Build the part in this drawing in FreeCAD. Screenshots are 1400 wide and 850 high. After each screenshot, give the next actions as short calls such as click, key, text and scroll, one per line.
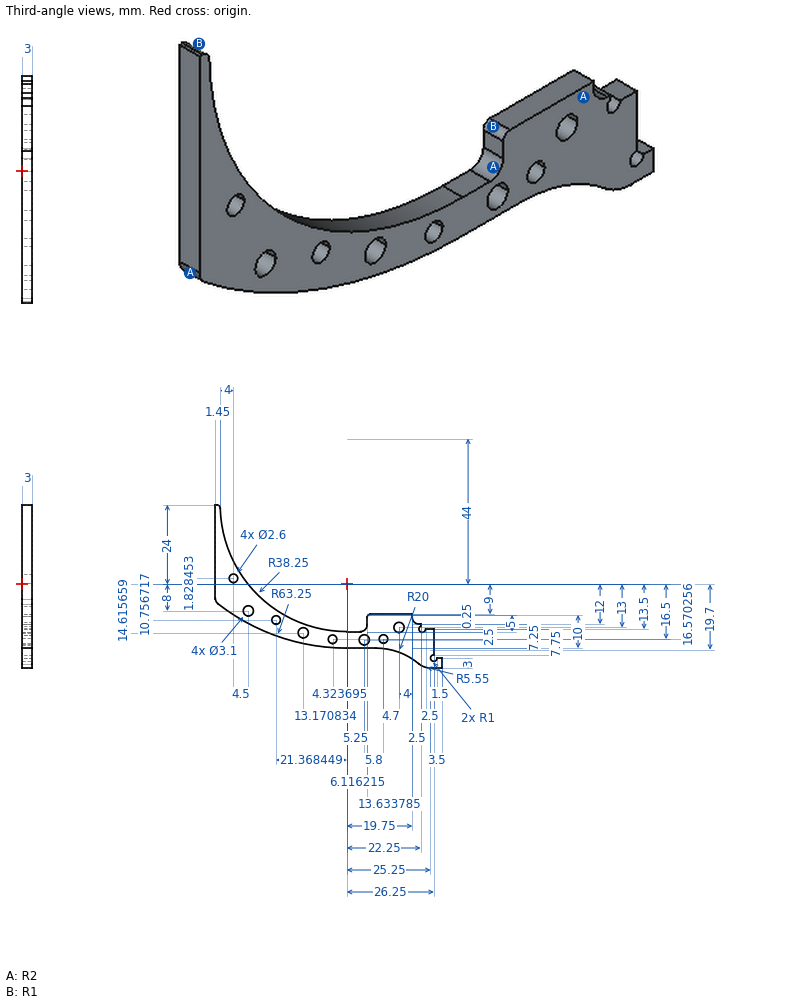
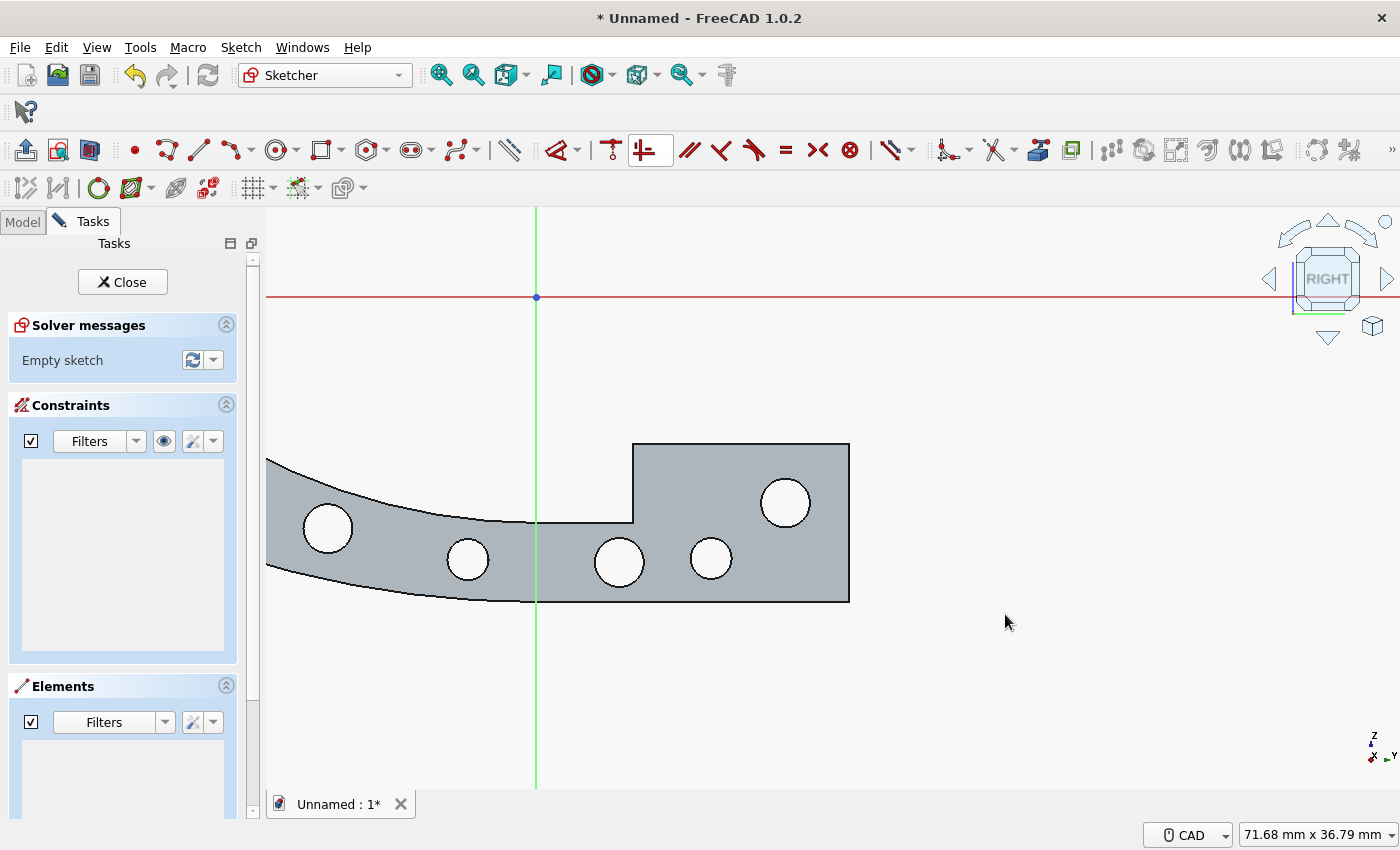
key(g)
key(r)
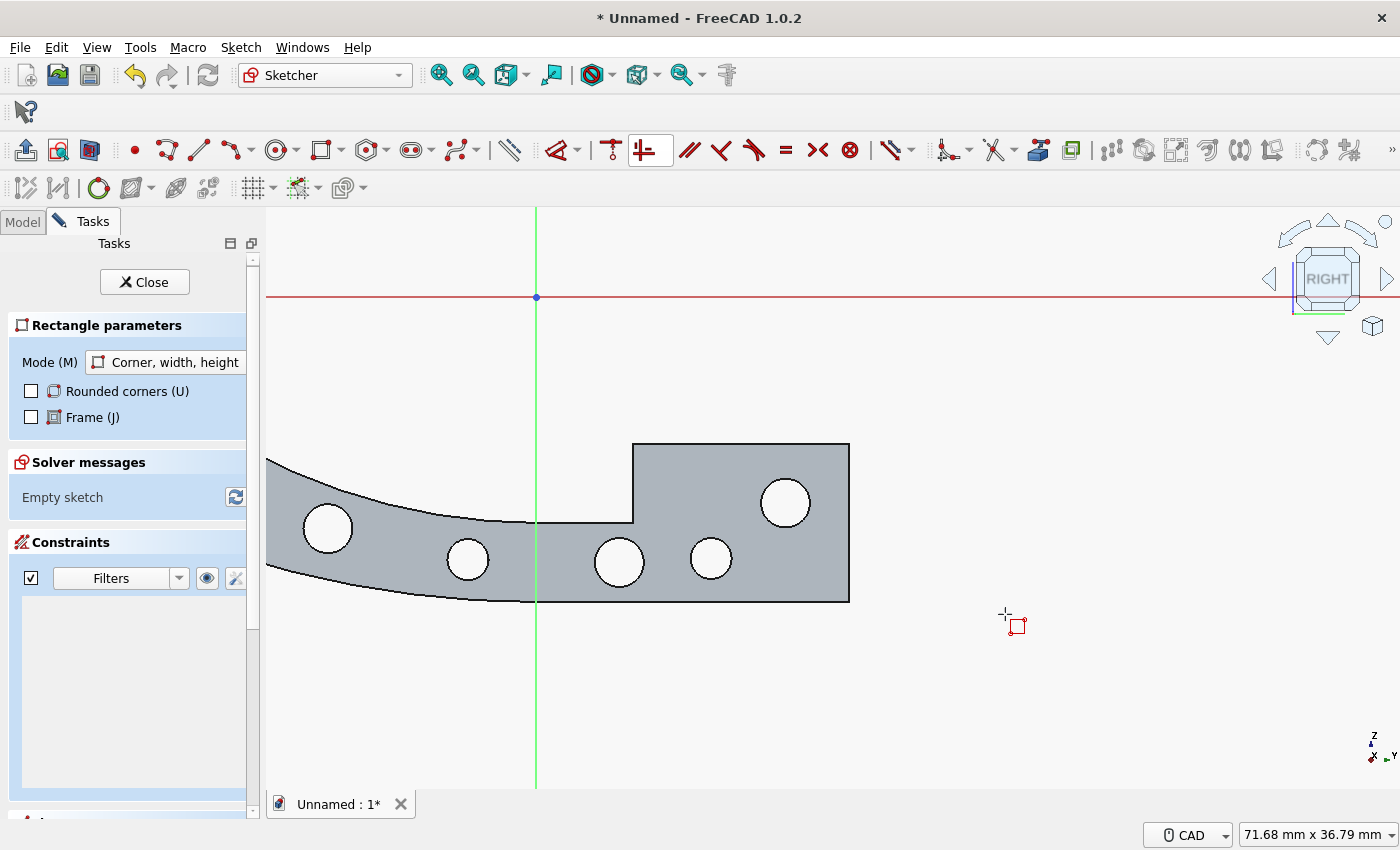
scroll(633, 440, up, 7)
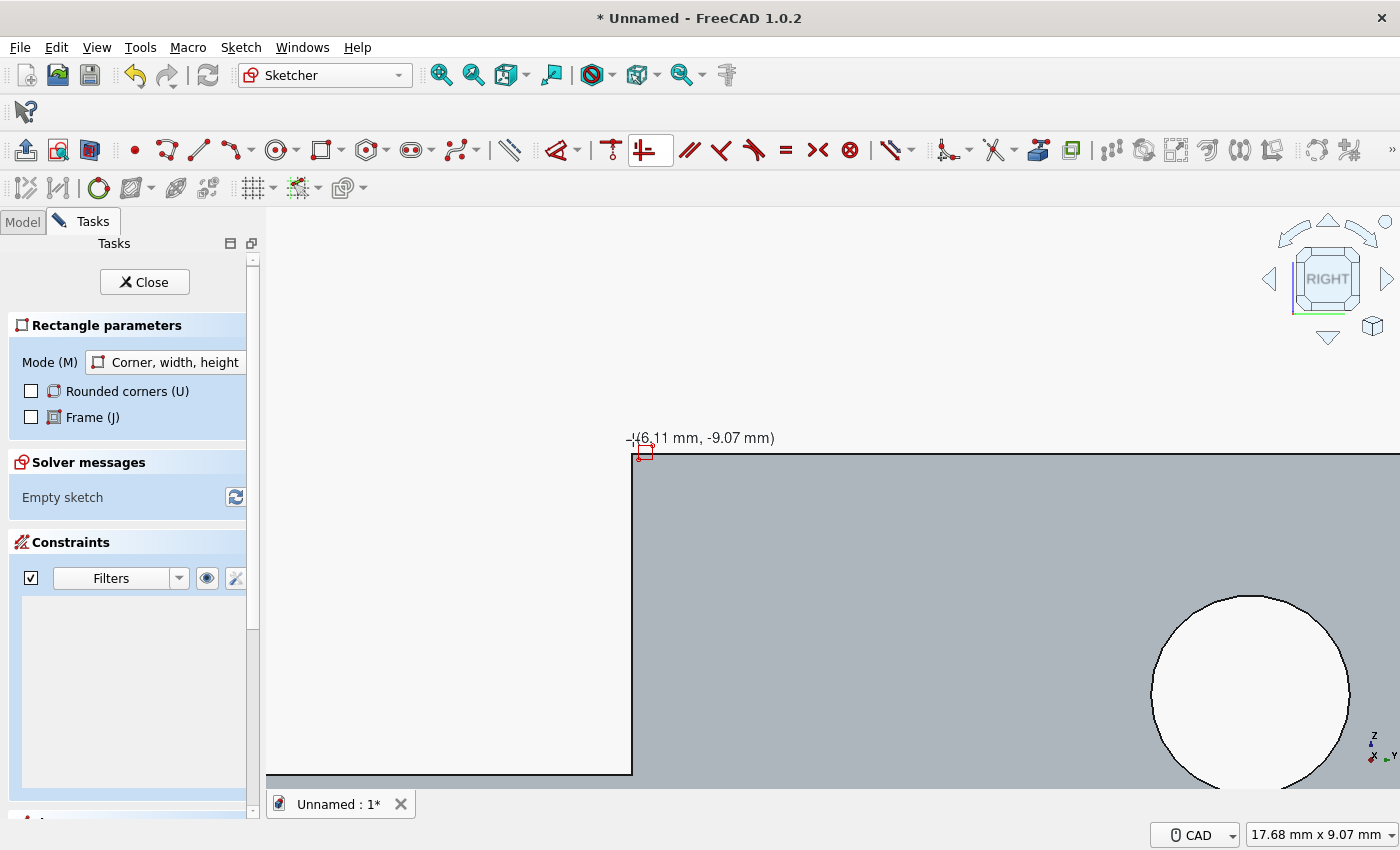
scroll(634, 441, down, 7)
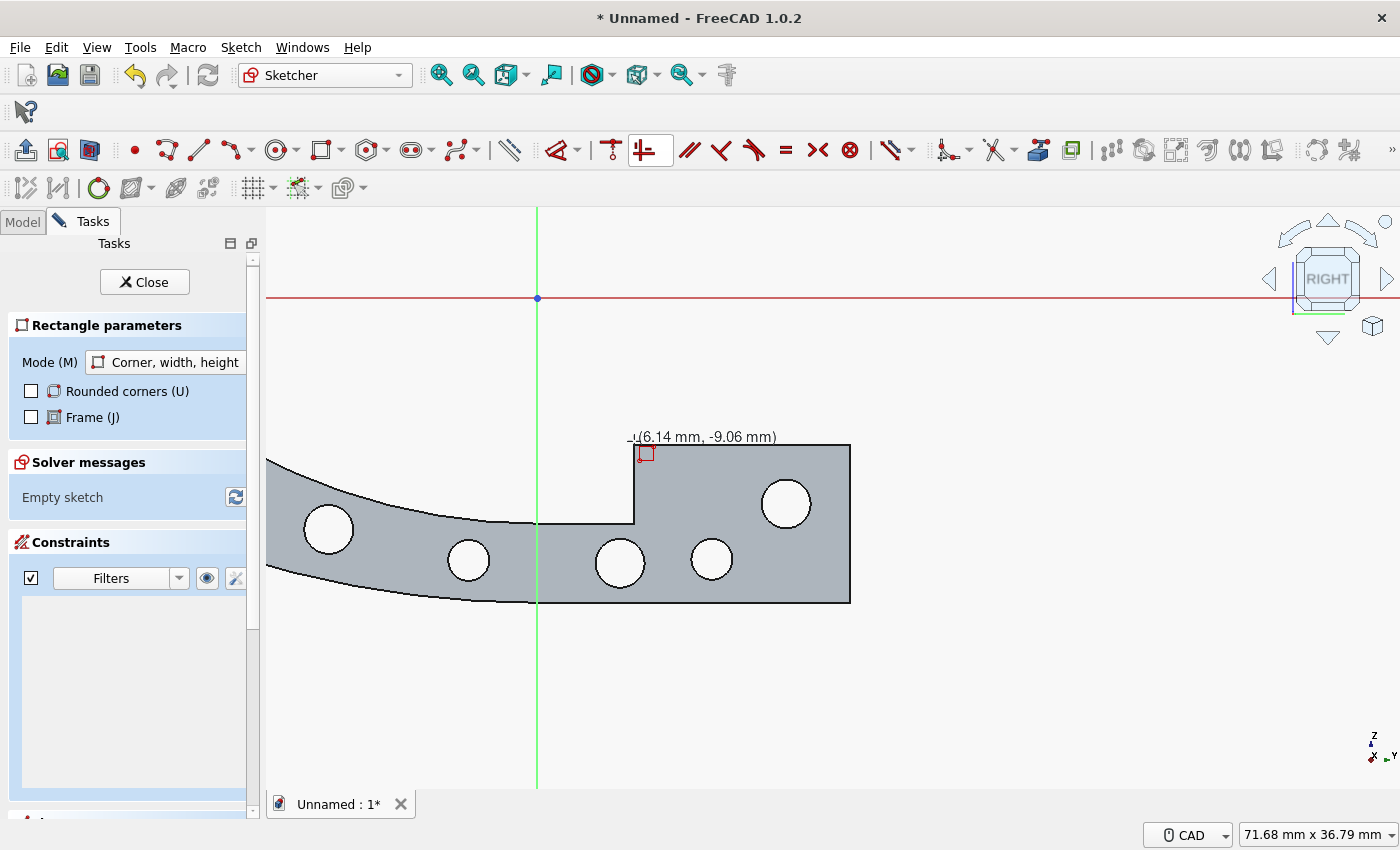
click(634, 441)
click(850, 445)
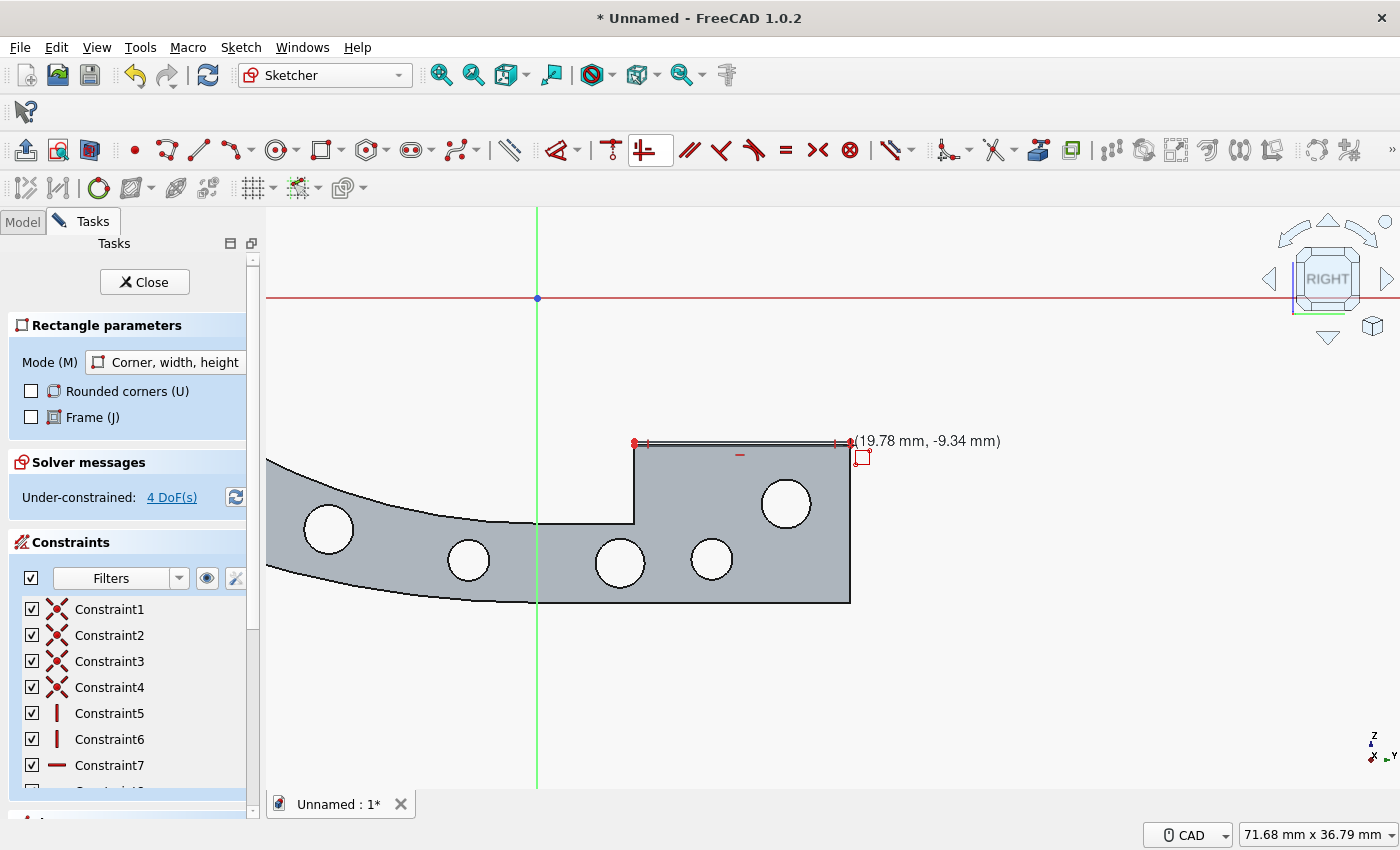
click(168, 150)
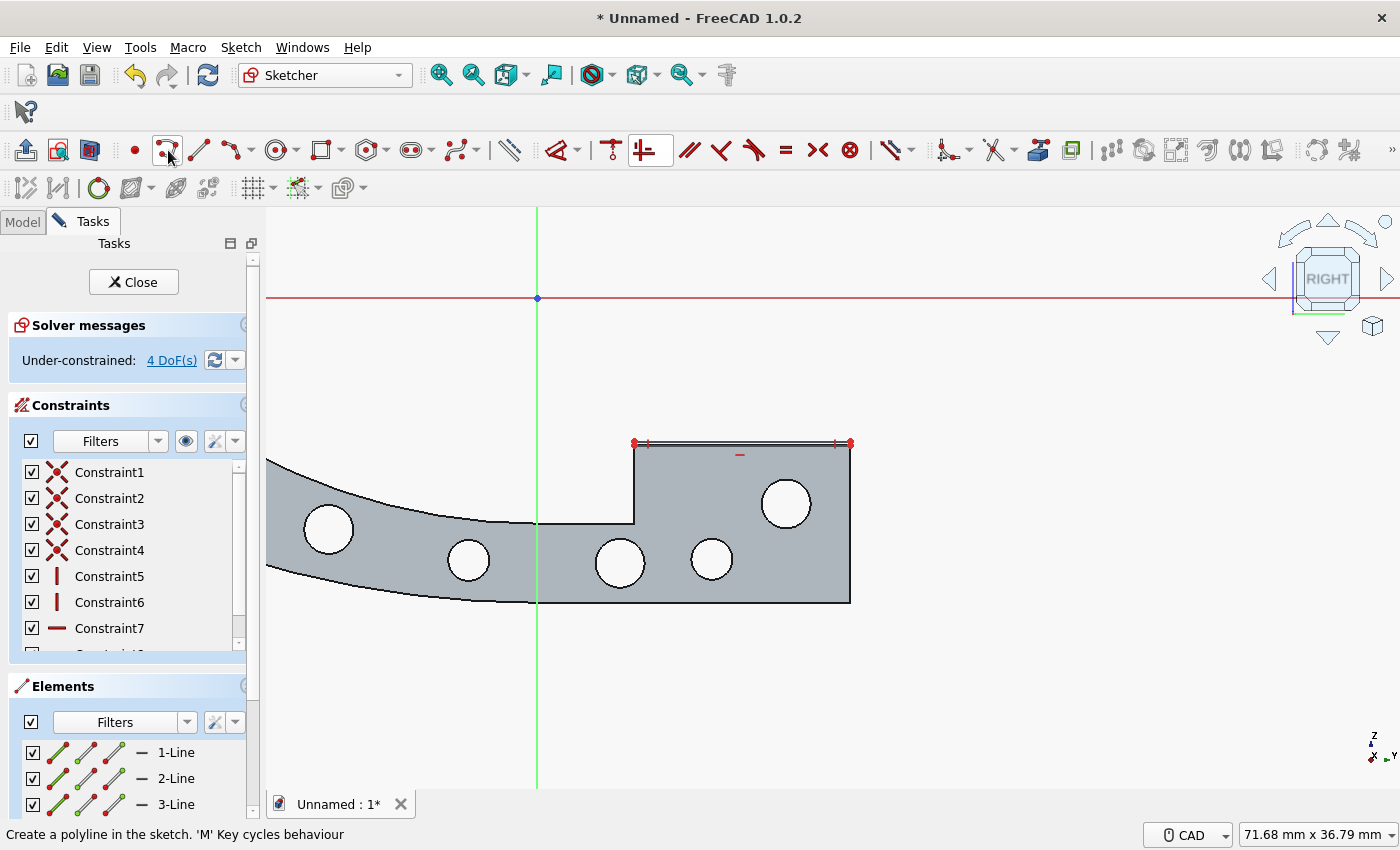
click(937, 698)
click(992, 698)
click(992, 650)
click(968, 650)
right_click(968, 650)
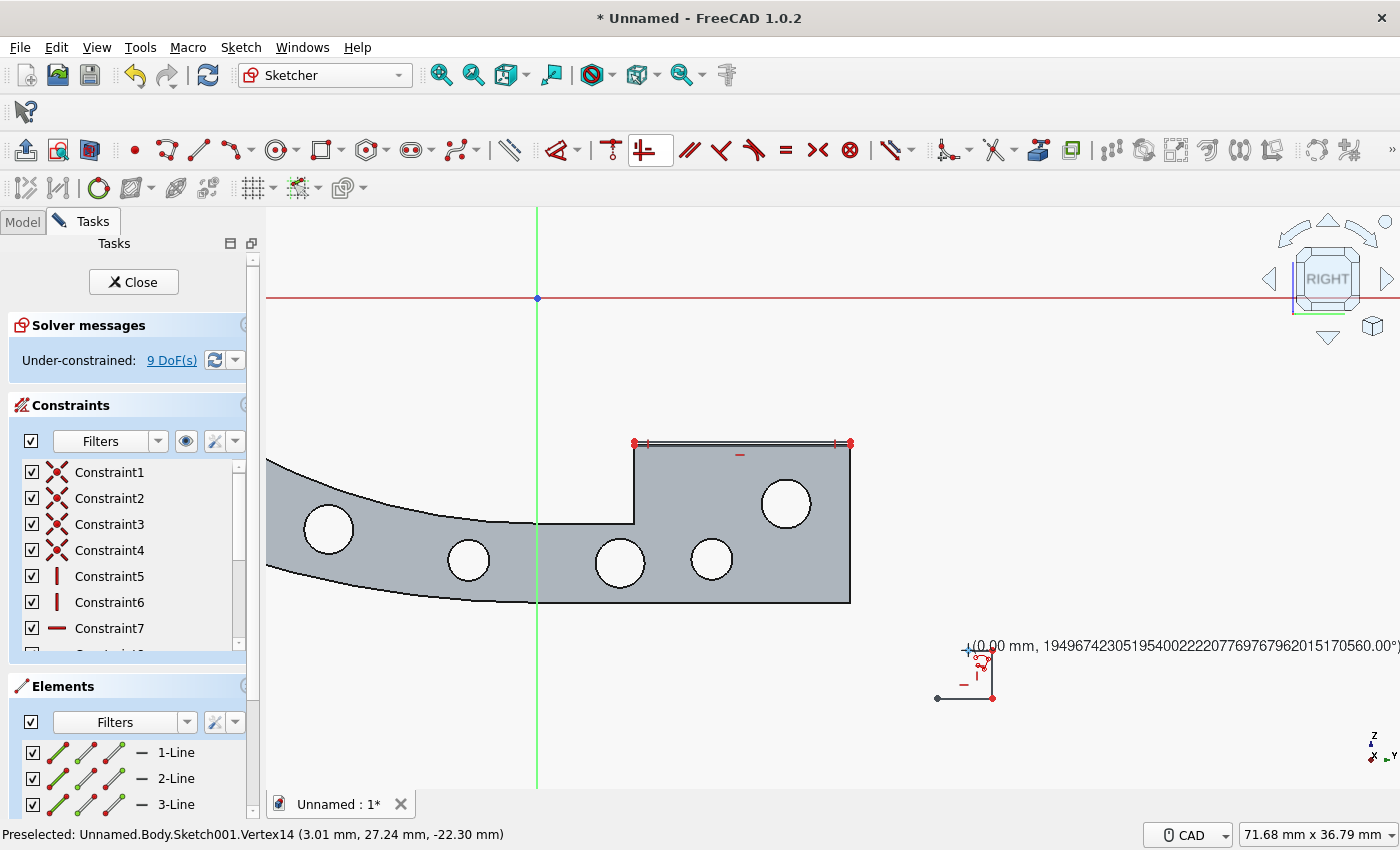
click(952, 634)
click(952, 512)
click(913, 512)
right_click(913, 512)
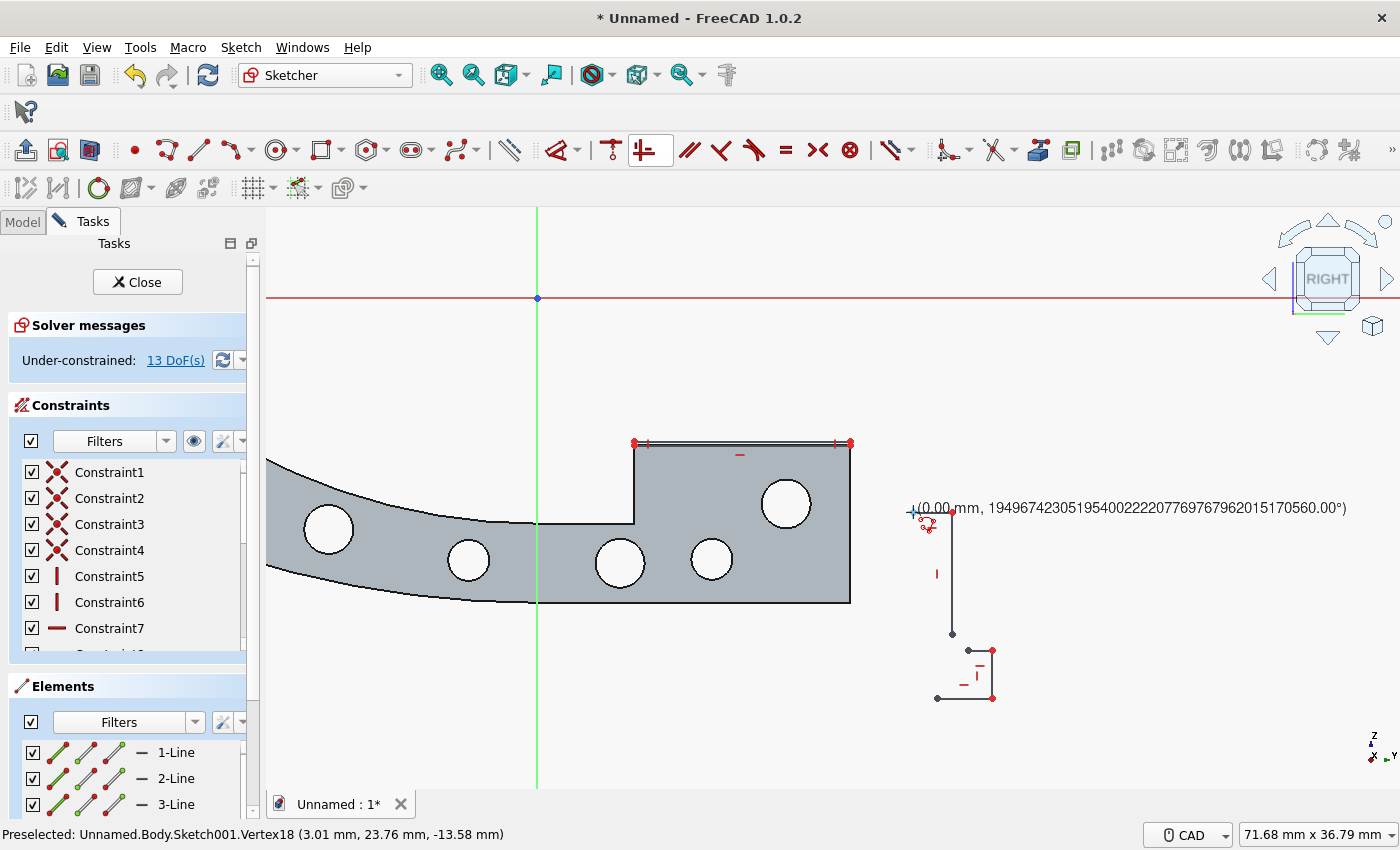
click(889, 498)